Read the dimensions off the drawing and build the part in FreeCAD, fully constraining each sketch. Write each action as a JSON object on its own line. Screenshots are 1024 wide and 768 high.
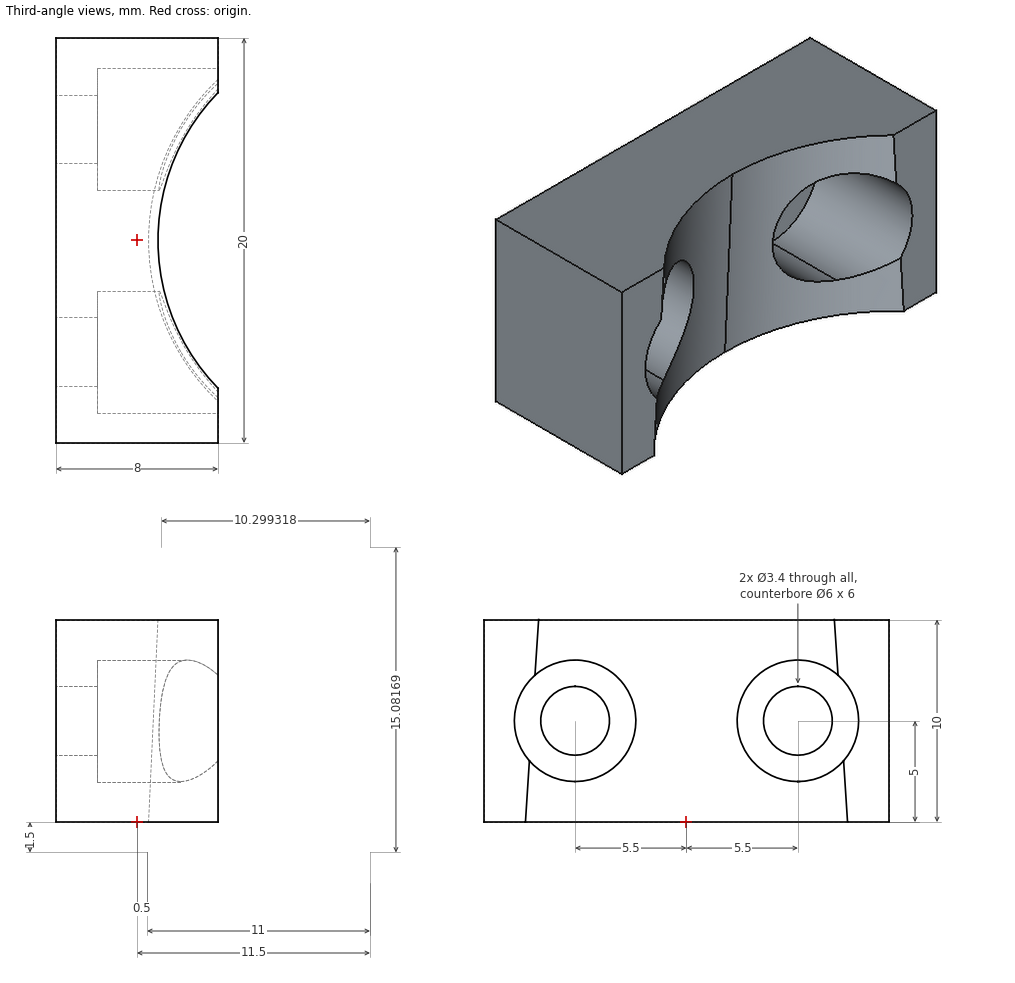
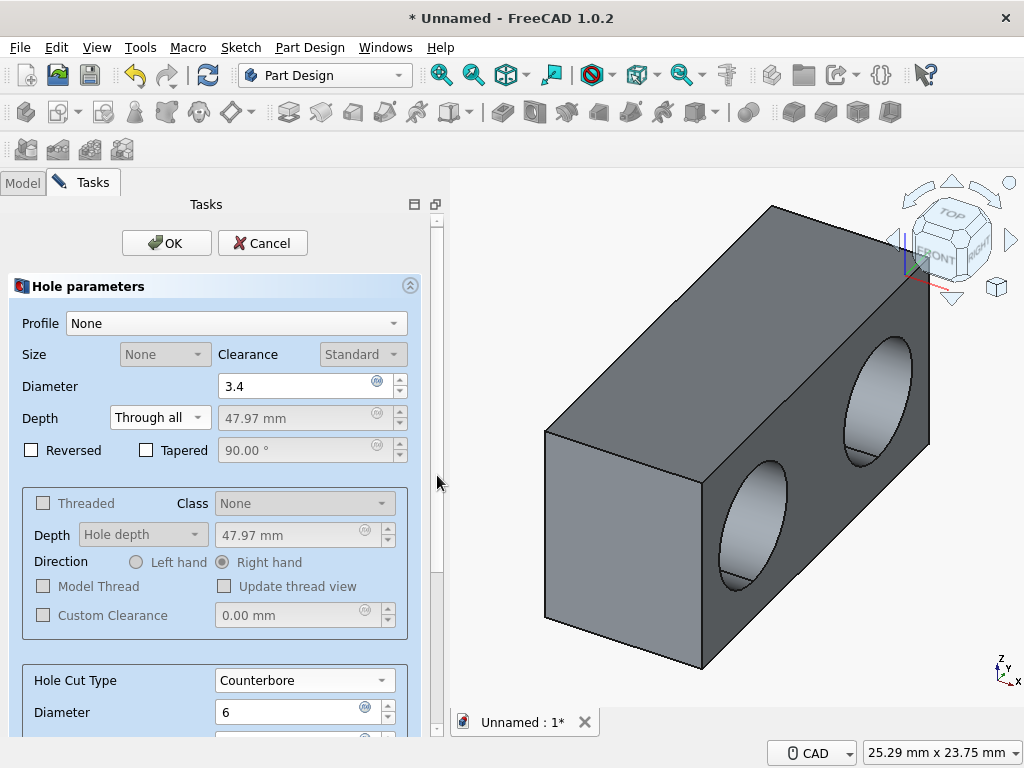
{"action": "left_click", "coordinate": [167, 243]}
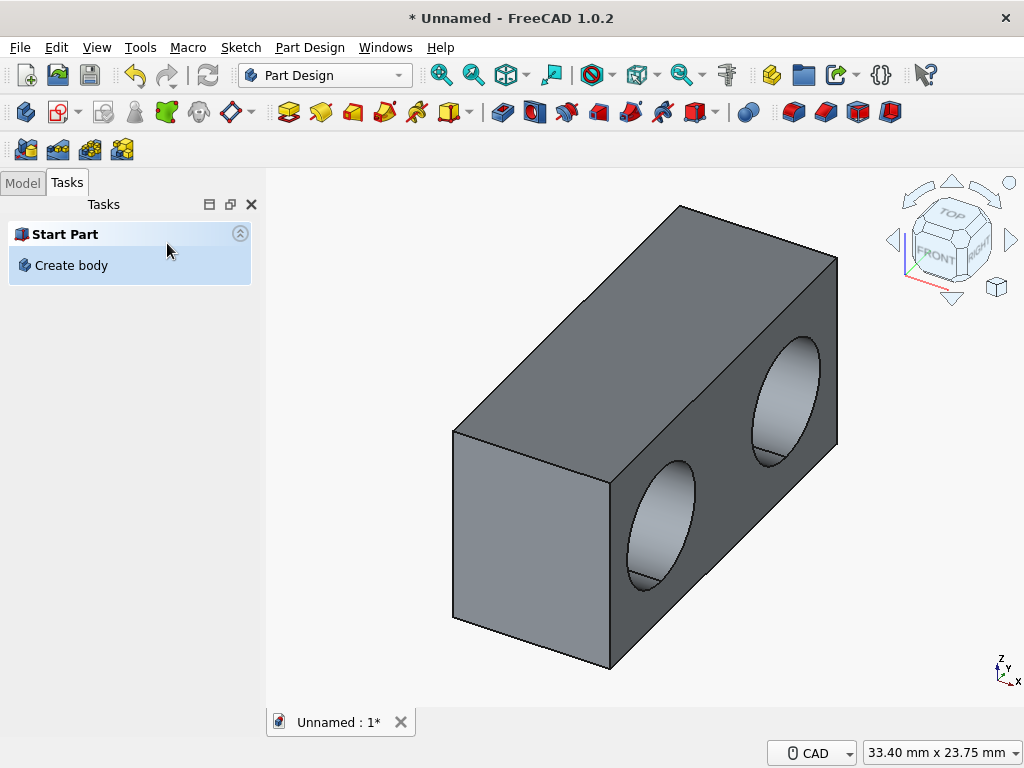
{"action": "left_click", "coordinate": [58, 112]}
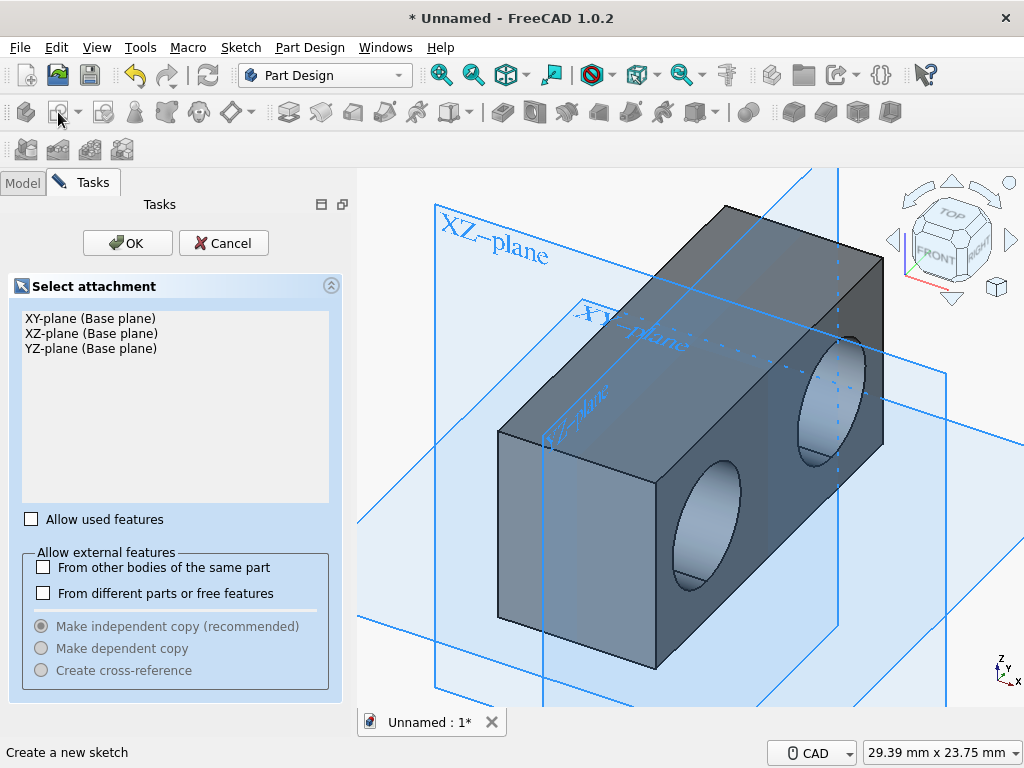
{"action": "left_click", "coordinate": [82, 334]}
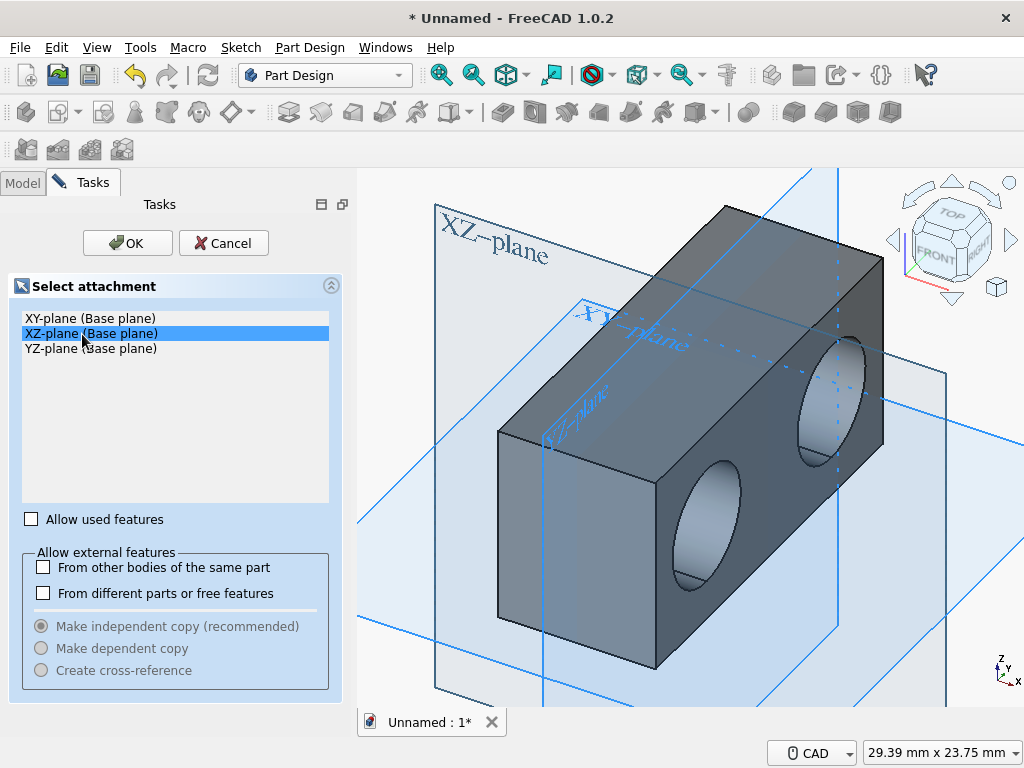
{"action": "left_click", "coordinate": [128, 243]}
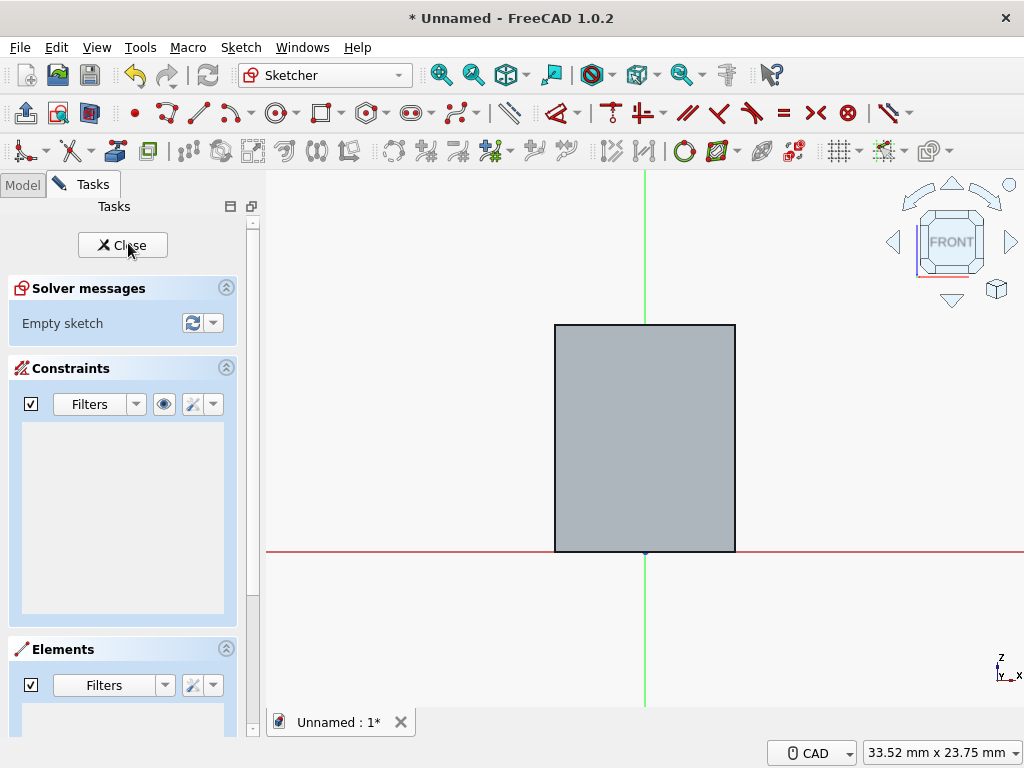
{"action": "left_click", "coordinate": [90, 114]}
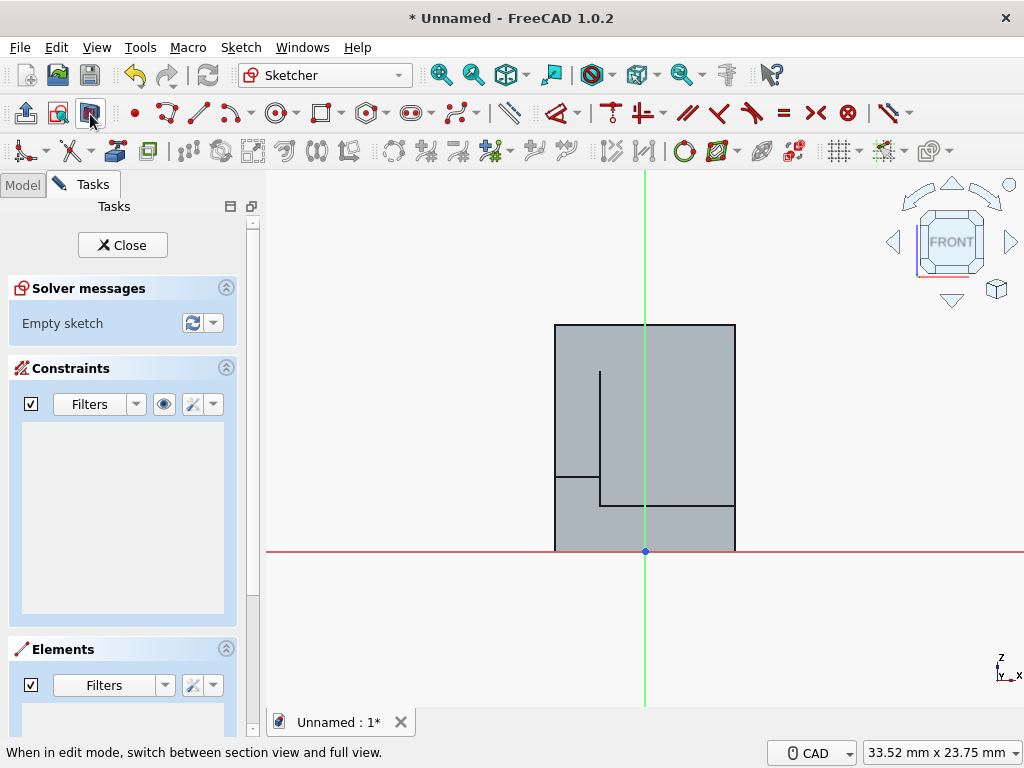
{"action": "scroll", "coordinate": [294, 348], "scroll_direction": "down", "scroll_amount": 2}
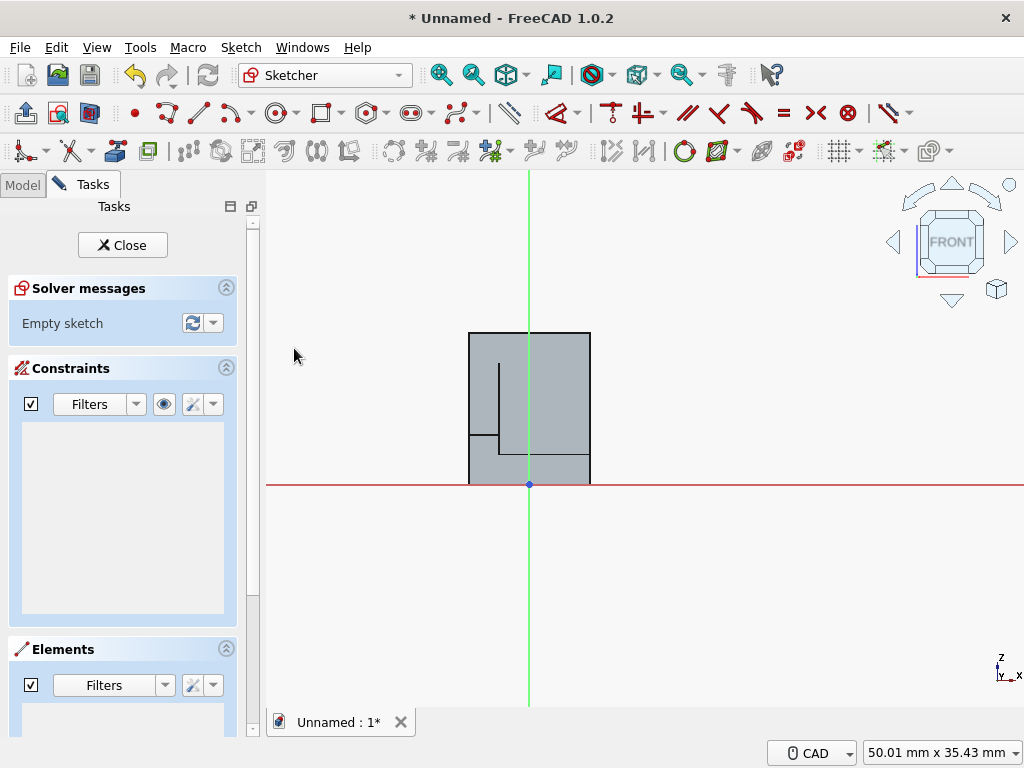
{"action": "key", "text": "g m"}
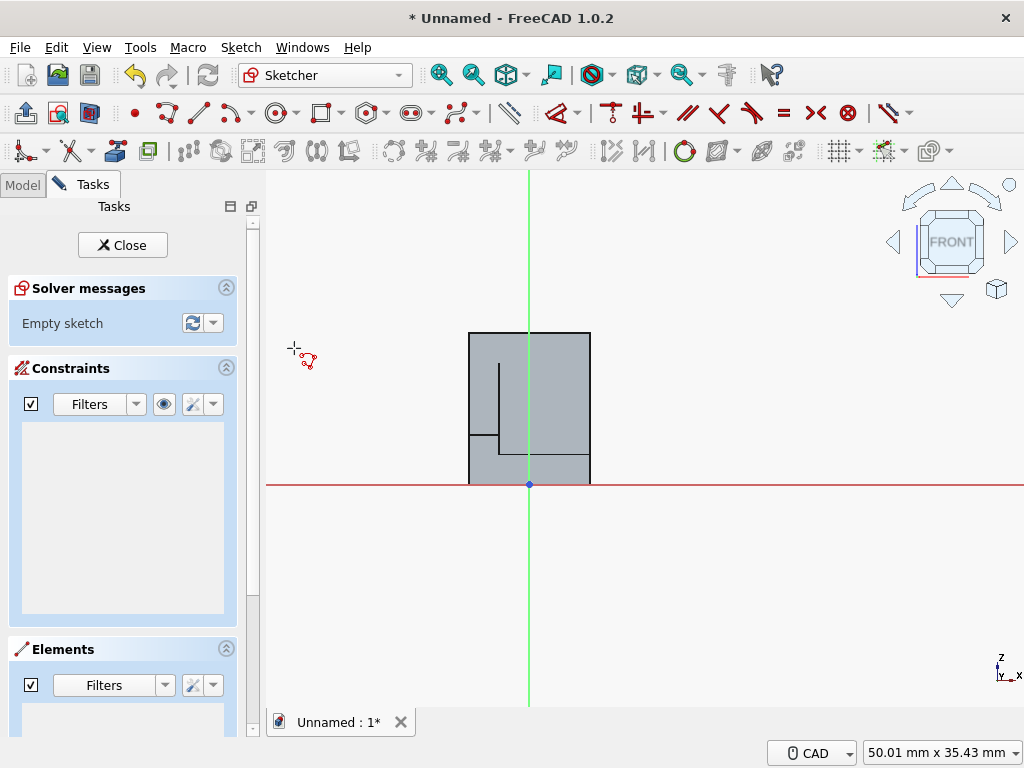
{"action": "scroll", "coordinate": [537, 507], "scroll_direction": "up", "scroll_amount": 4}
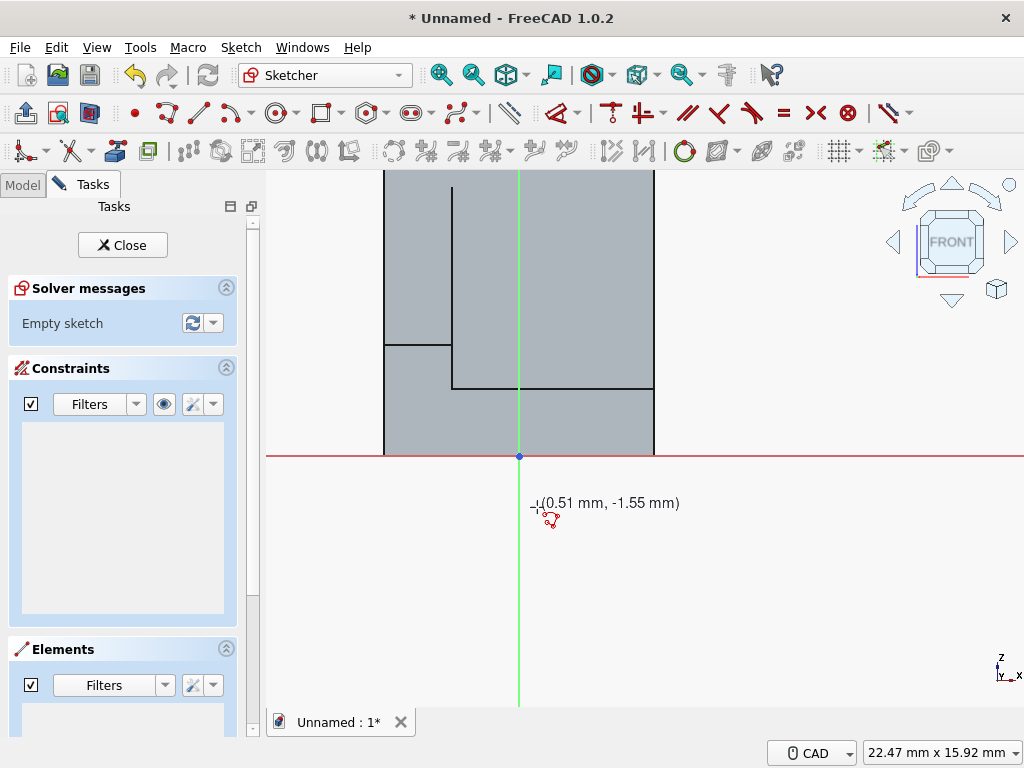
{"action": "left_click", "coordinate": [536, 507]}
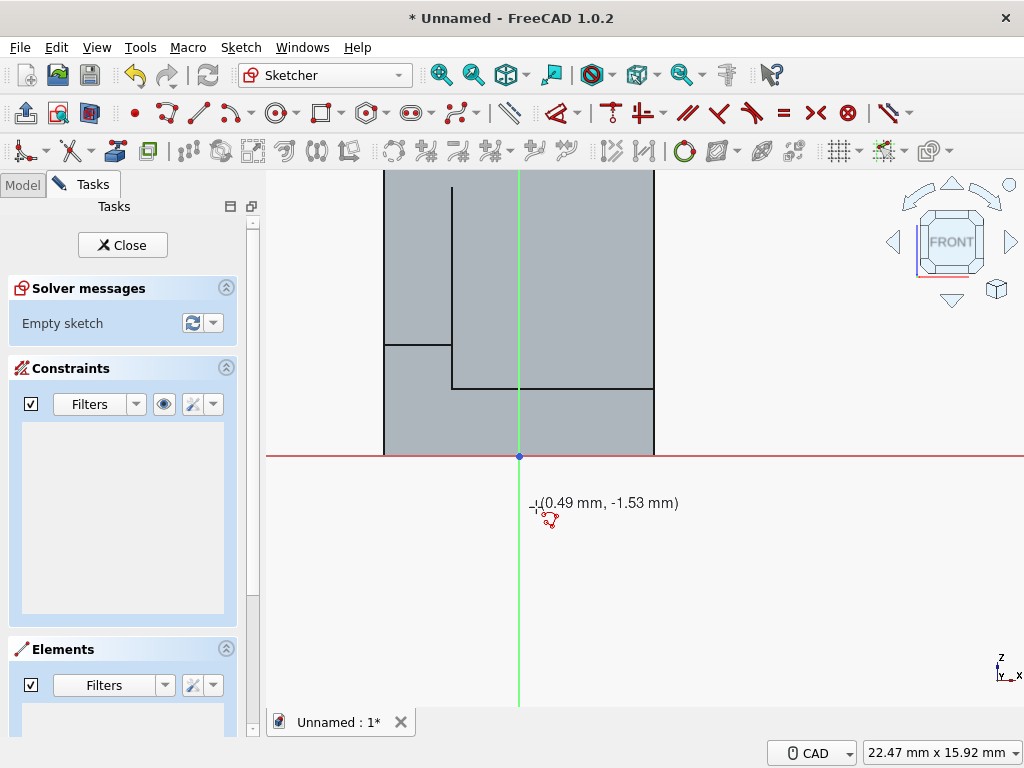
{"action": "scroll", "coordinate": [465, 507], "scroll_direction": "down", "scroll_amount": 4}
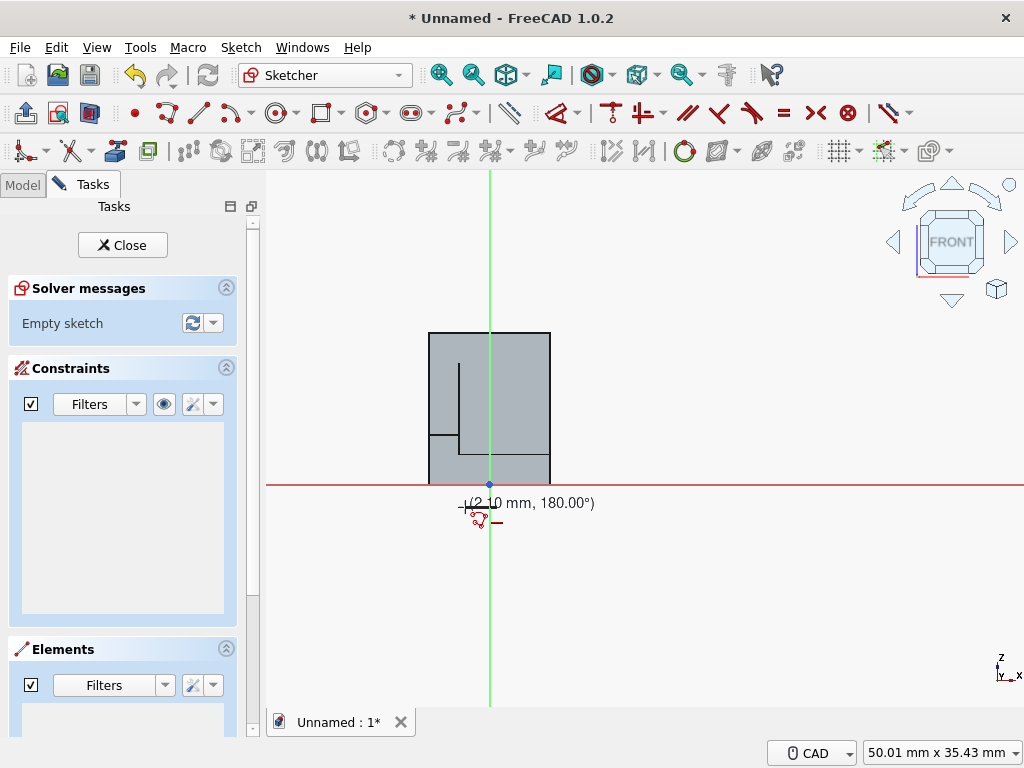
{"action": "left_click", "coordinate": [509, 279]}
{"action": "left_click", "coordinate": [664, 279]}
{"action": "left_click", "coordinate": [664, 507]}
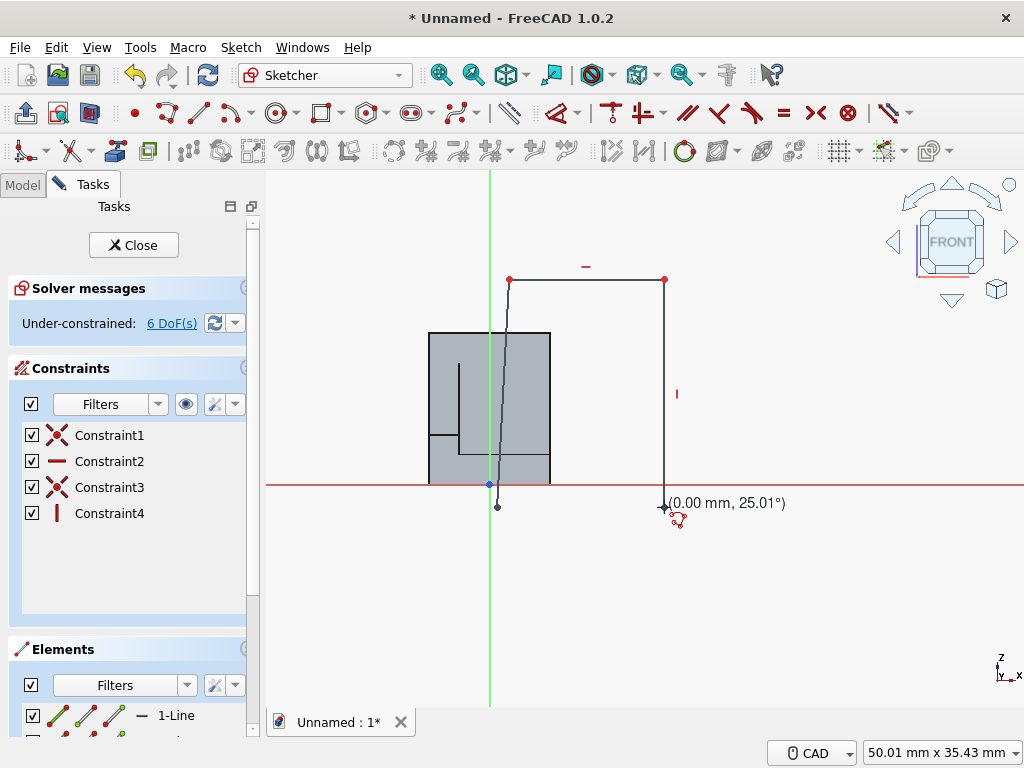
{"action": "scroll", "coordinate": [497, 507], "scroll_direction": "up", "scroll_amount": 4}